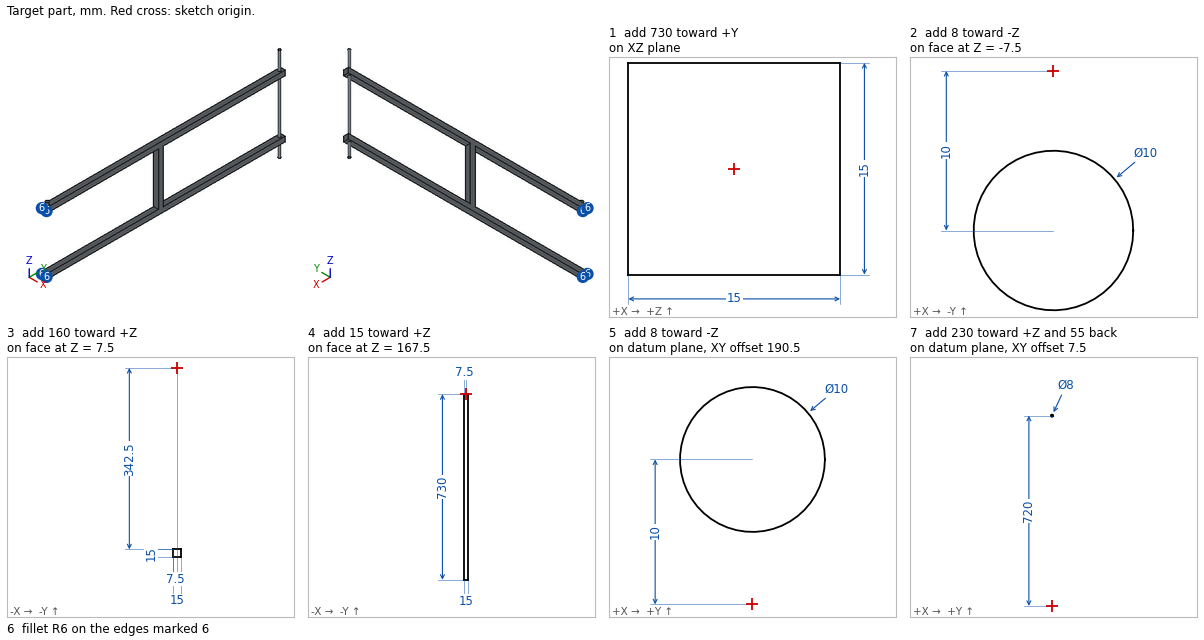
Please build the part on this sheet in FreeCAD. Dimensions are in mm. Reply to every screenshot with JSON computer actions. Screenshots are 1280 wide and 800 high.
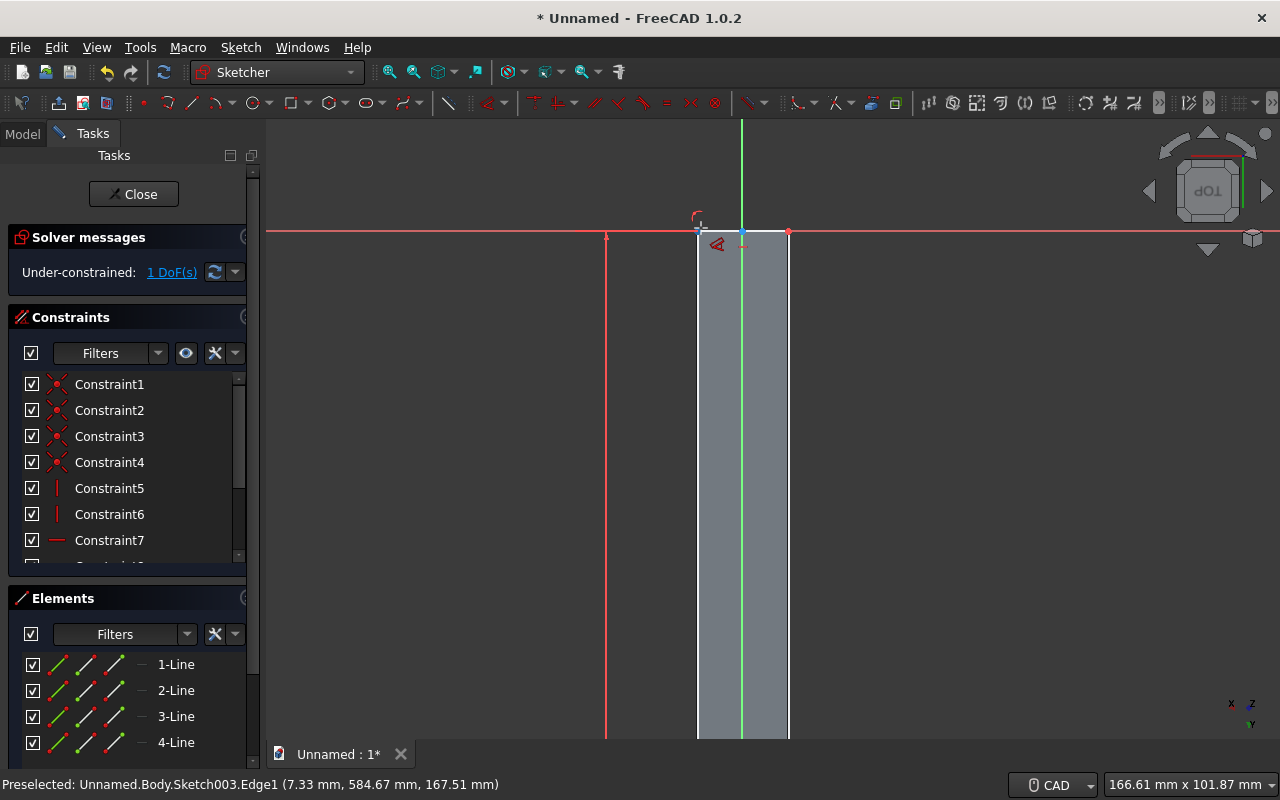
{"action": "left_click", "coordinate": [698, 231]}
{"action": "left_click", "coordinate": [720, 197]}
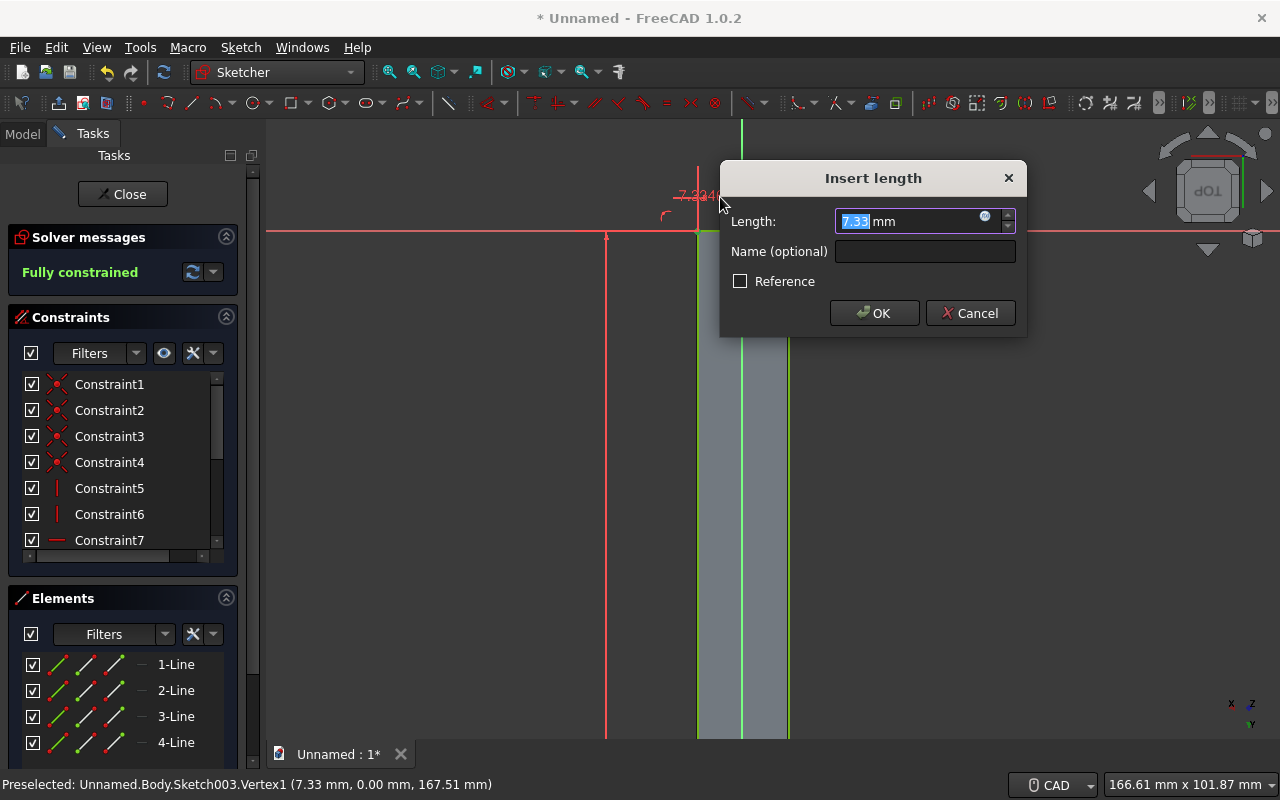
{"action": "type", "text": "7.5"}
{"action": "key", "text": "Return"}
{"action": "key", "text": "Escape"}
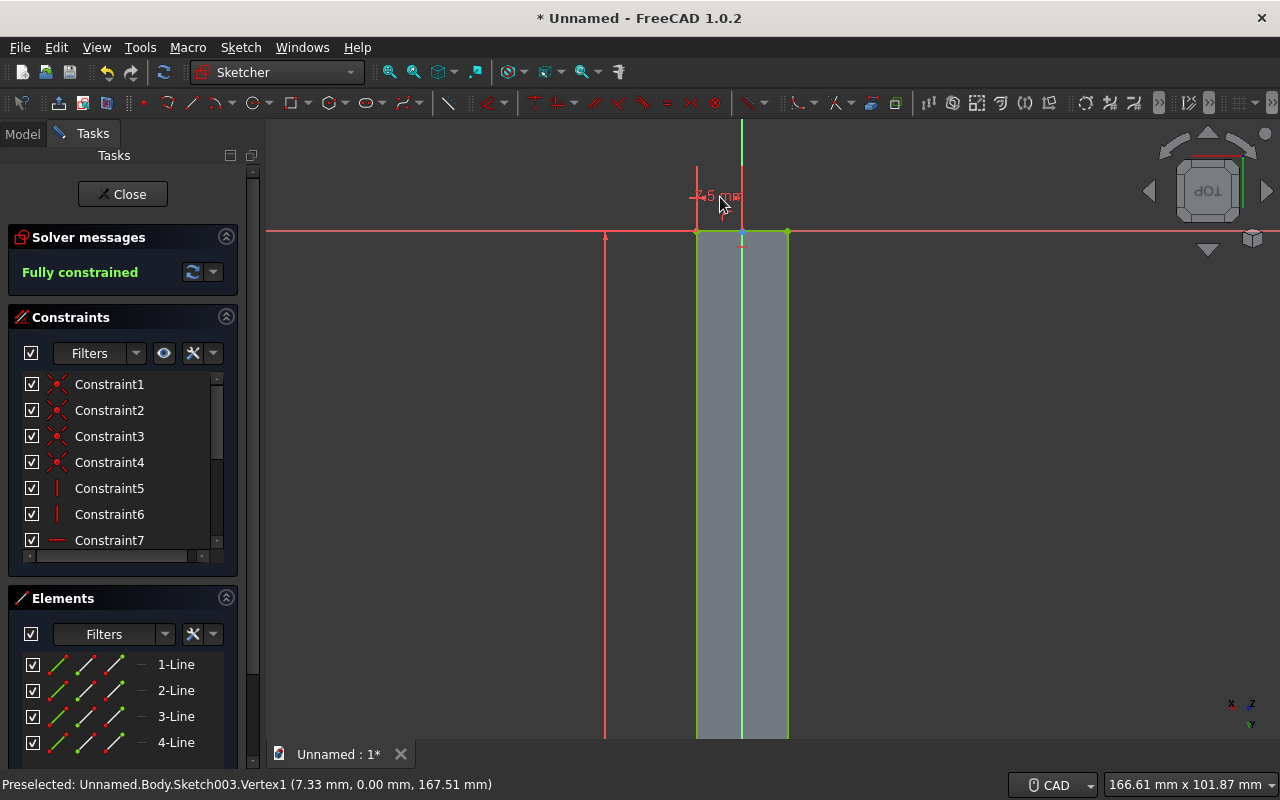
{"action": "left_click", "coordinate": [123, 194]}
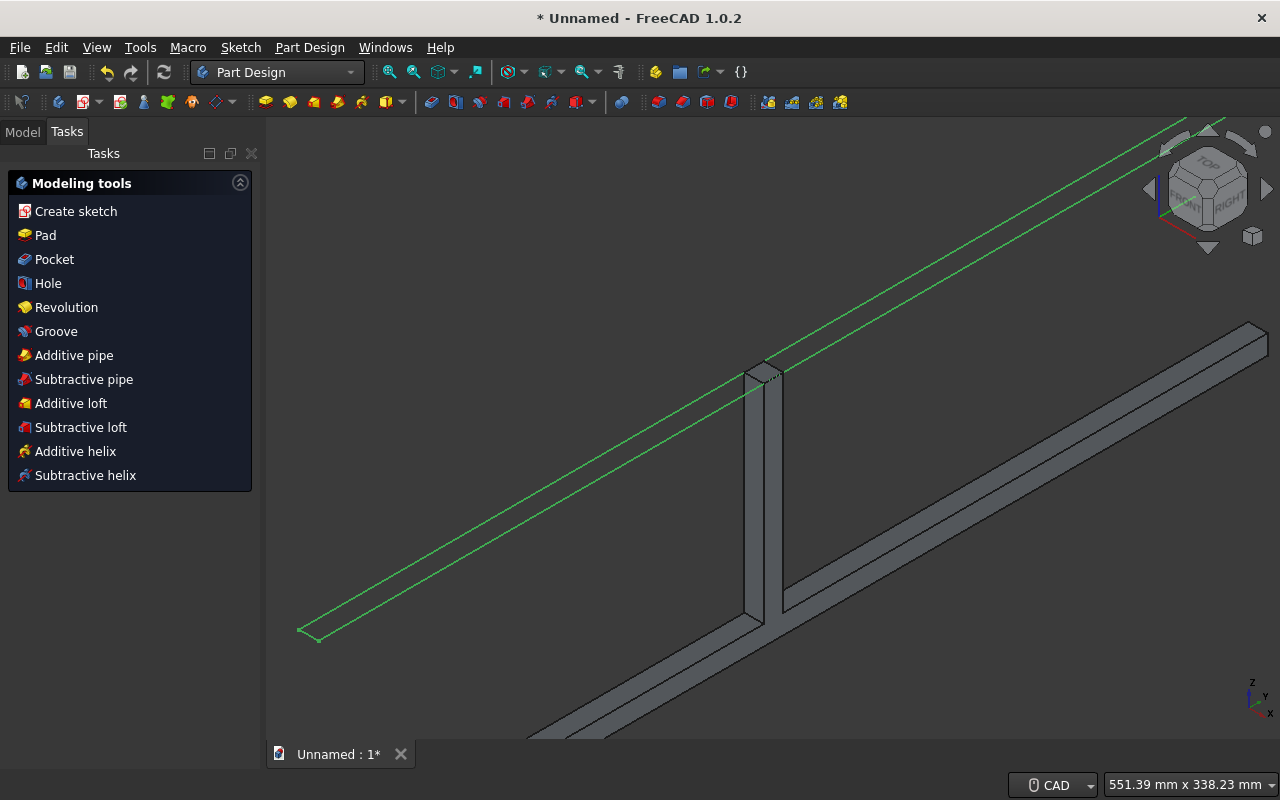
{"action": "left_click", "coordinate": [266, 102]}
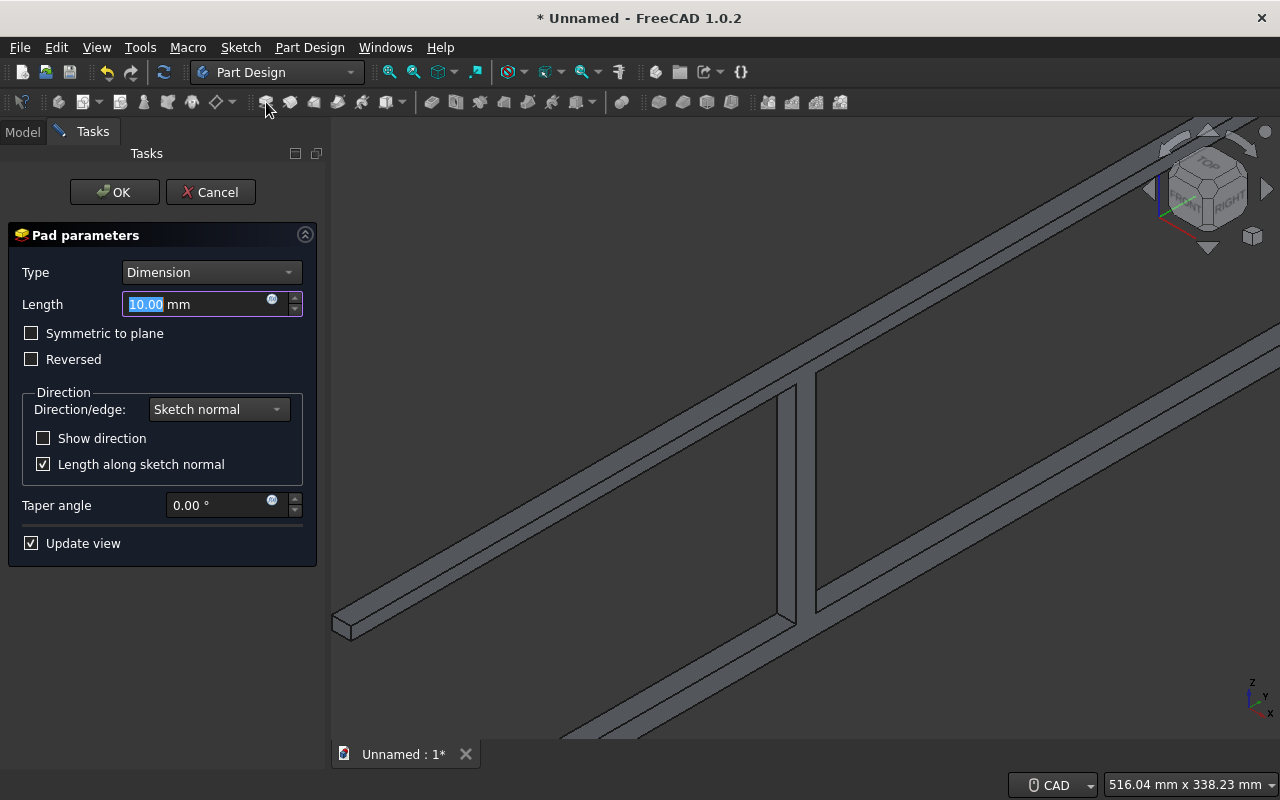
{"action": "type", "text": "15"}
{"action": "key", "text": "Tab"}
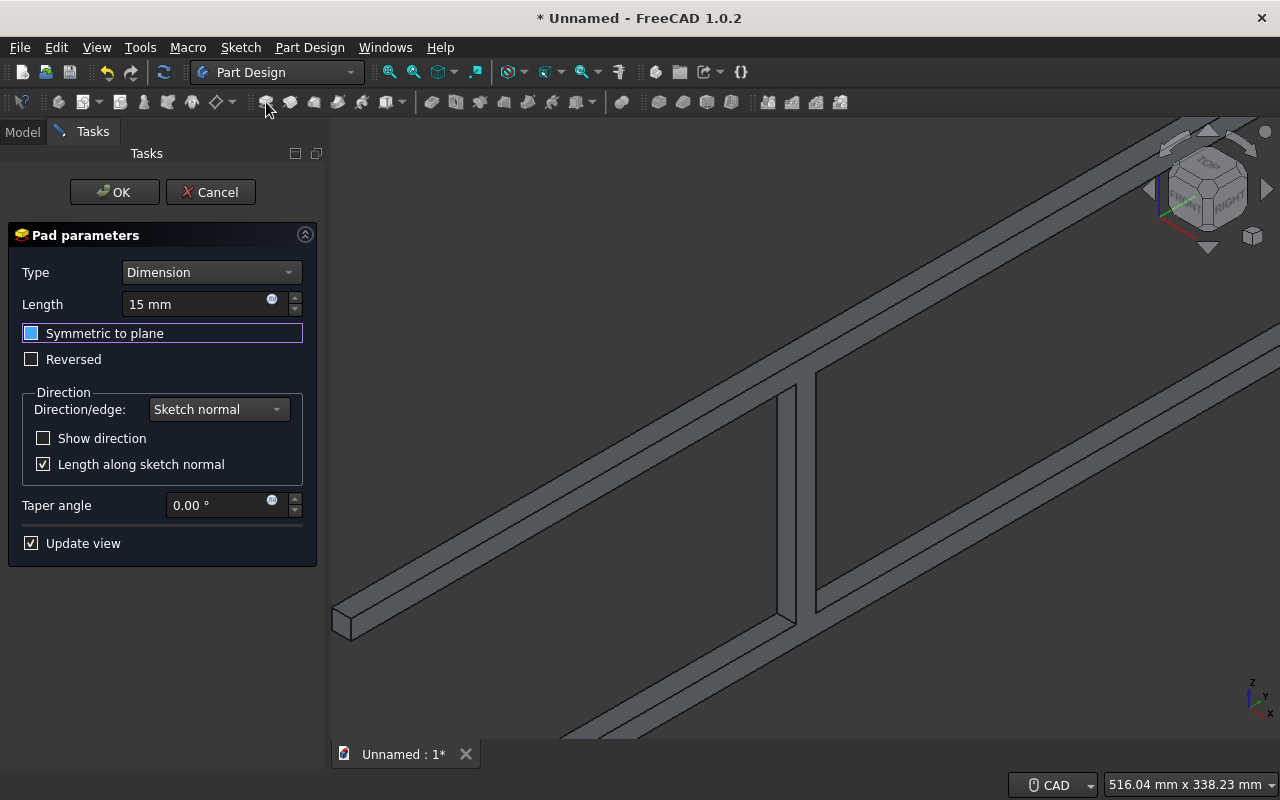
{"action": "left_click", "coordinate": [115, 192]}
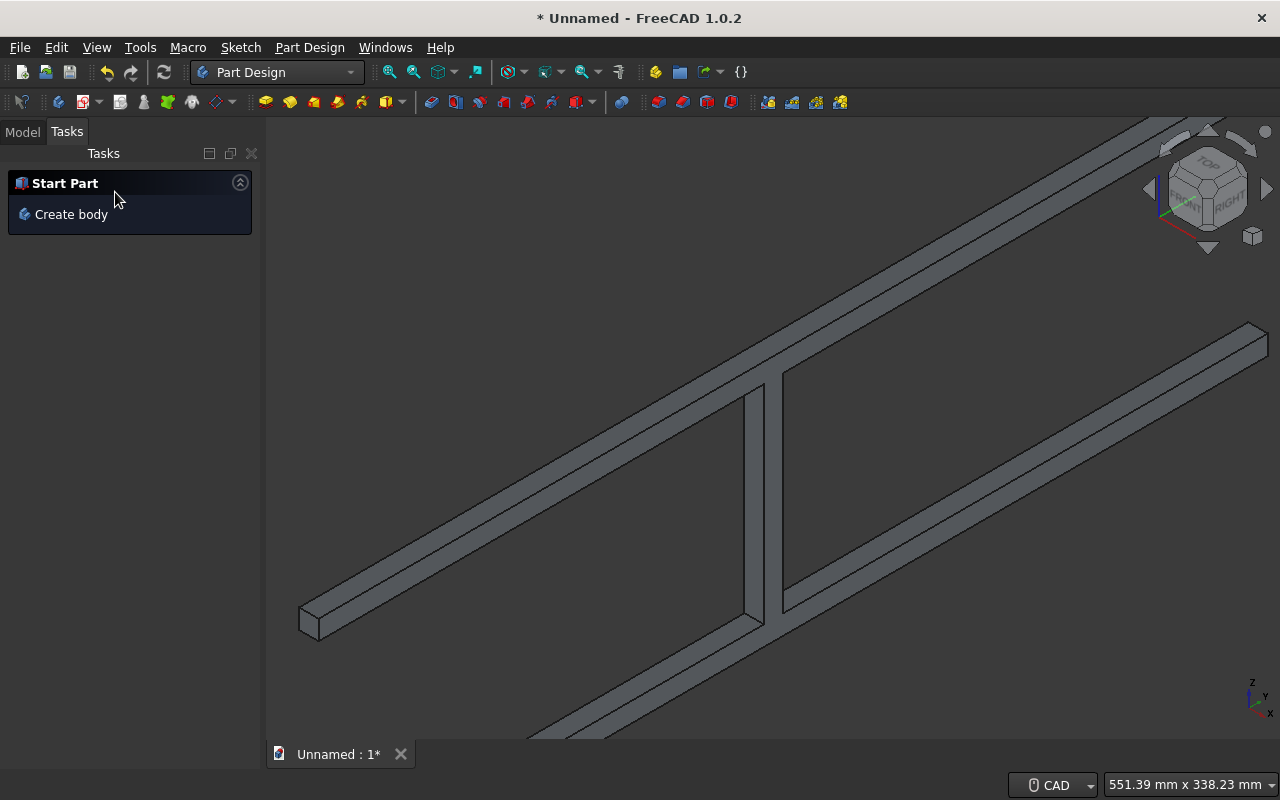
{"action": "left_click", "coordinate": [390, 72]}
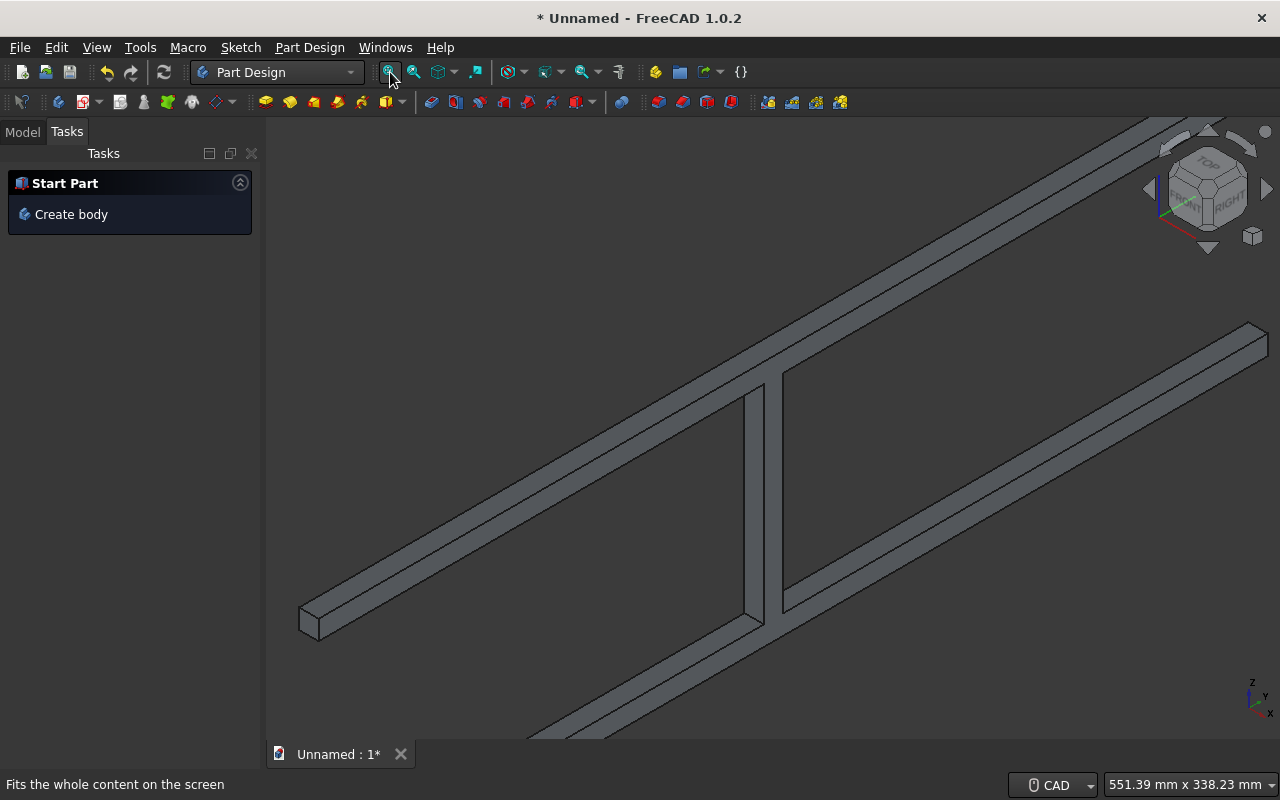
{"action": "left_click", "coordinate": [23, 131]}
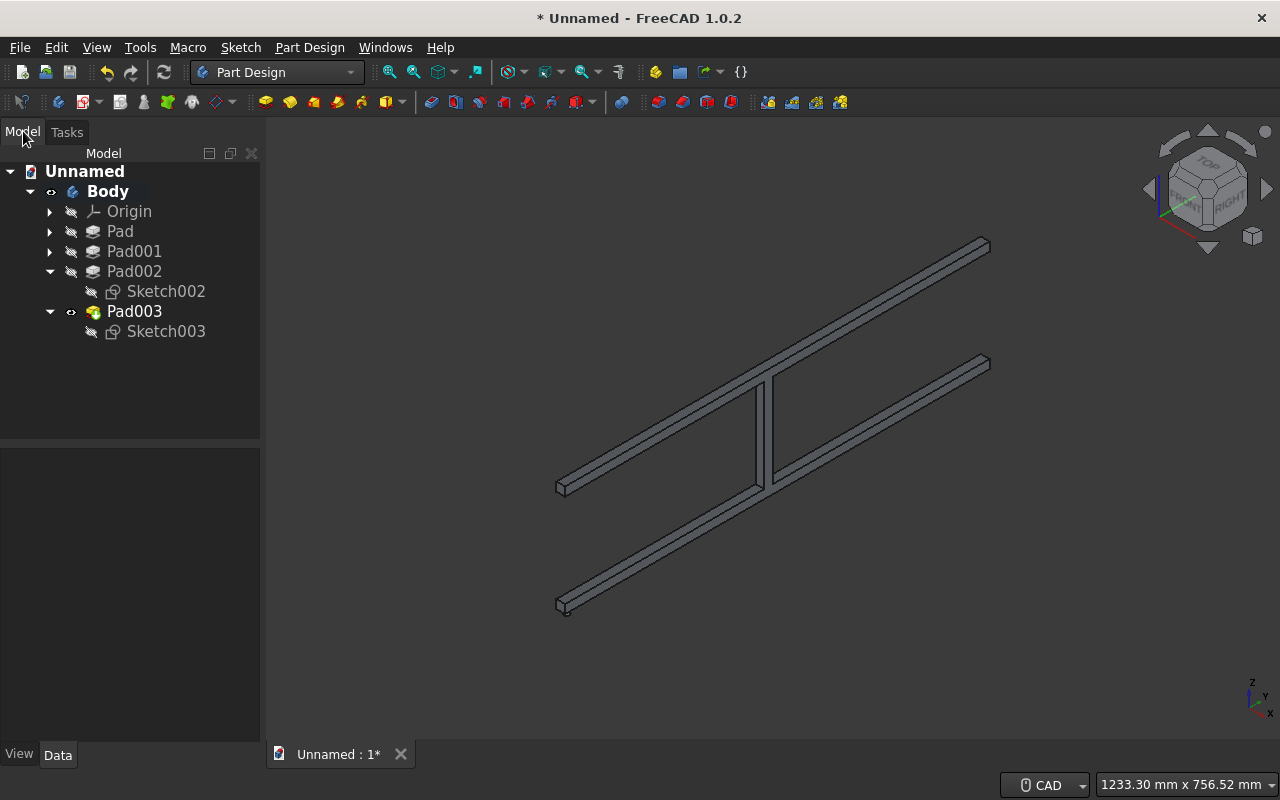
{"action": "left_click", "coordinate": [50, 212]}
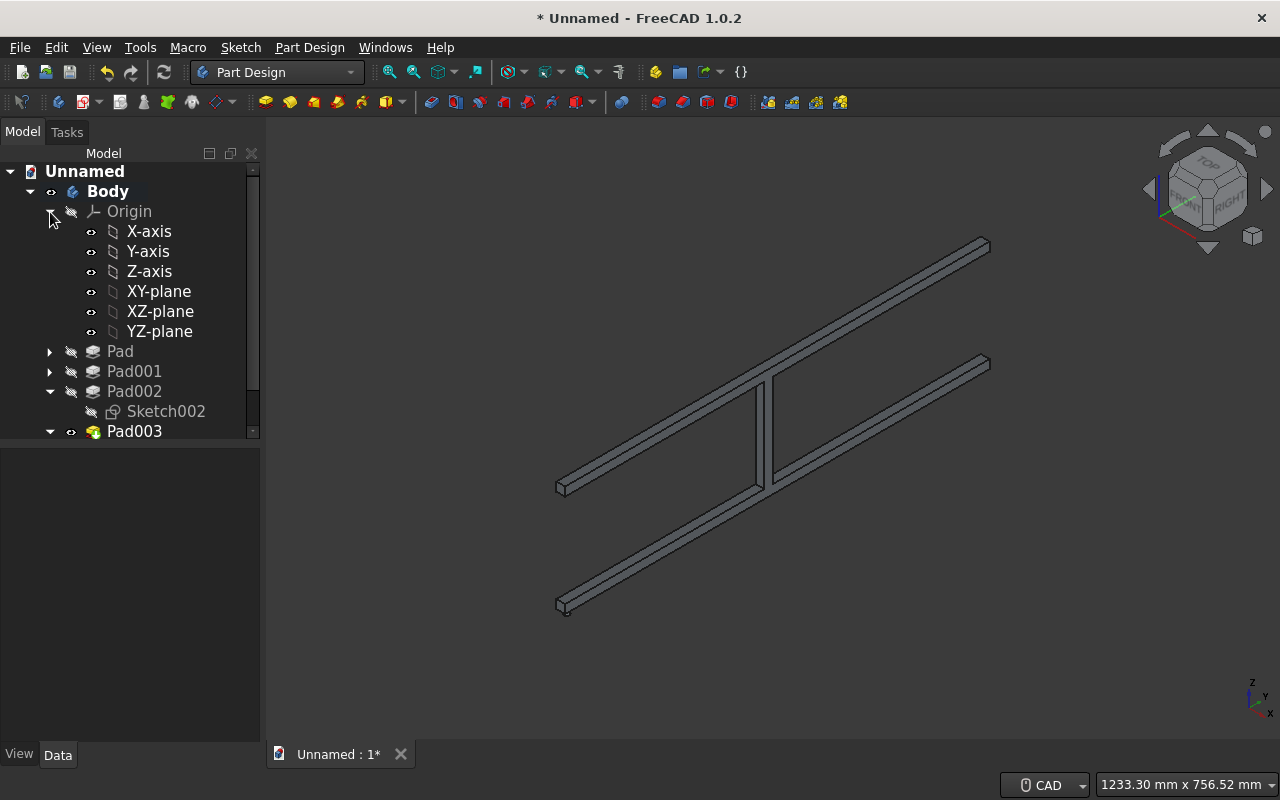
{"action": "left_click", "coordinate": [136, 292]}